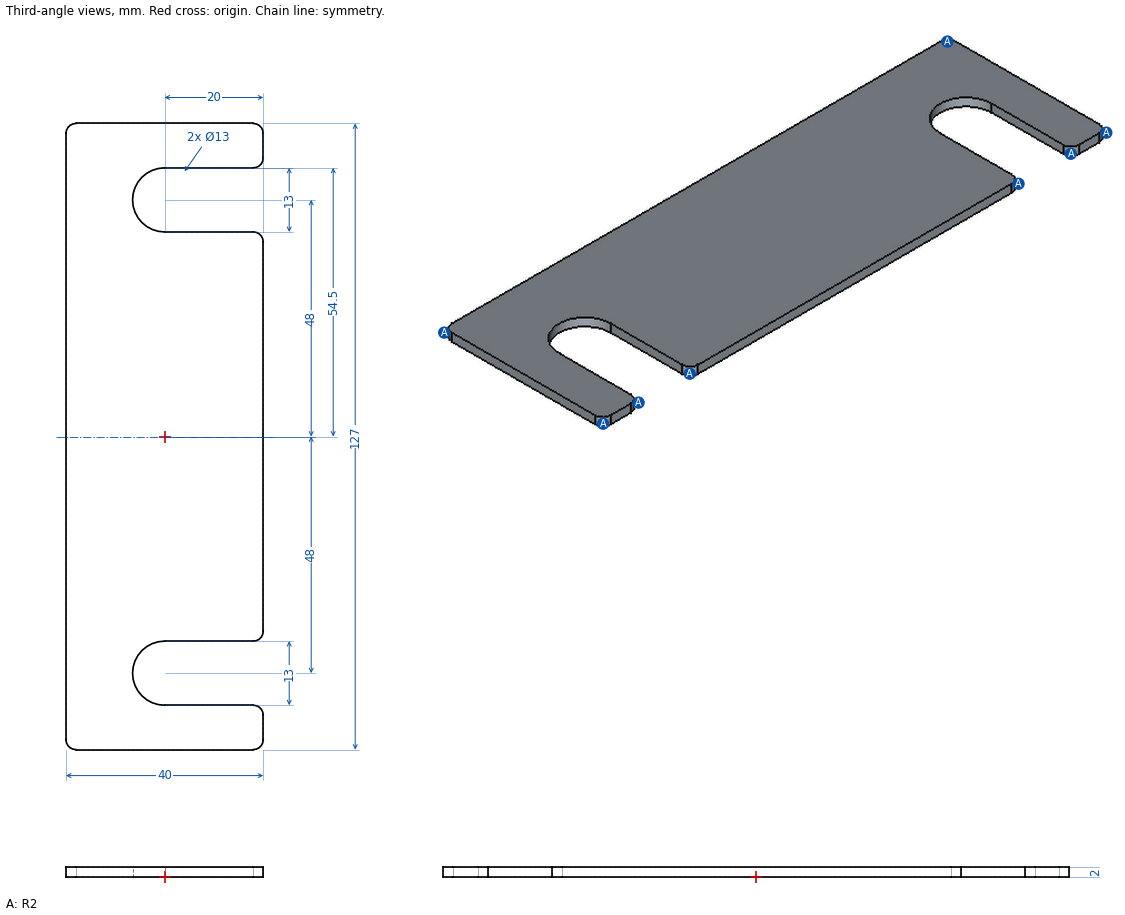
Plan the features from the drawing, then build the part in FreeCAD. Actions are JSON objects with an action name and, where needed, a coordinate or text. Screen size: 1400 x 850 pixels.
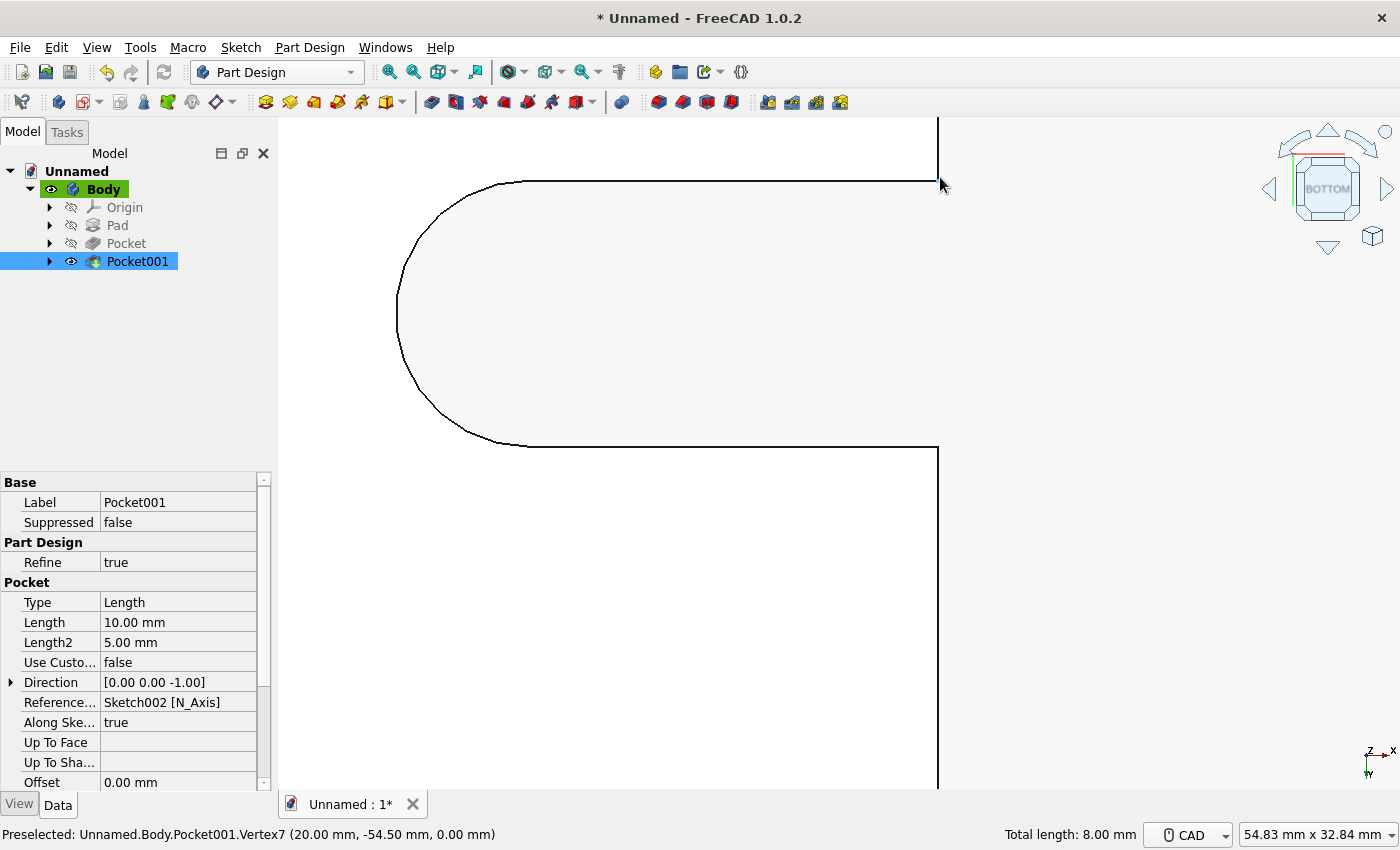
{"action": "left_click", "coordinate": [390, 72]}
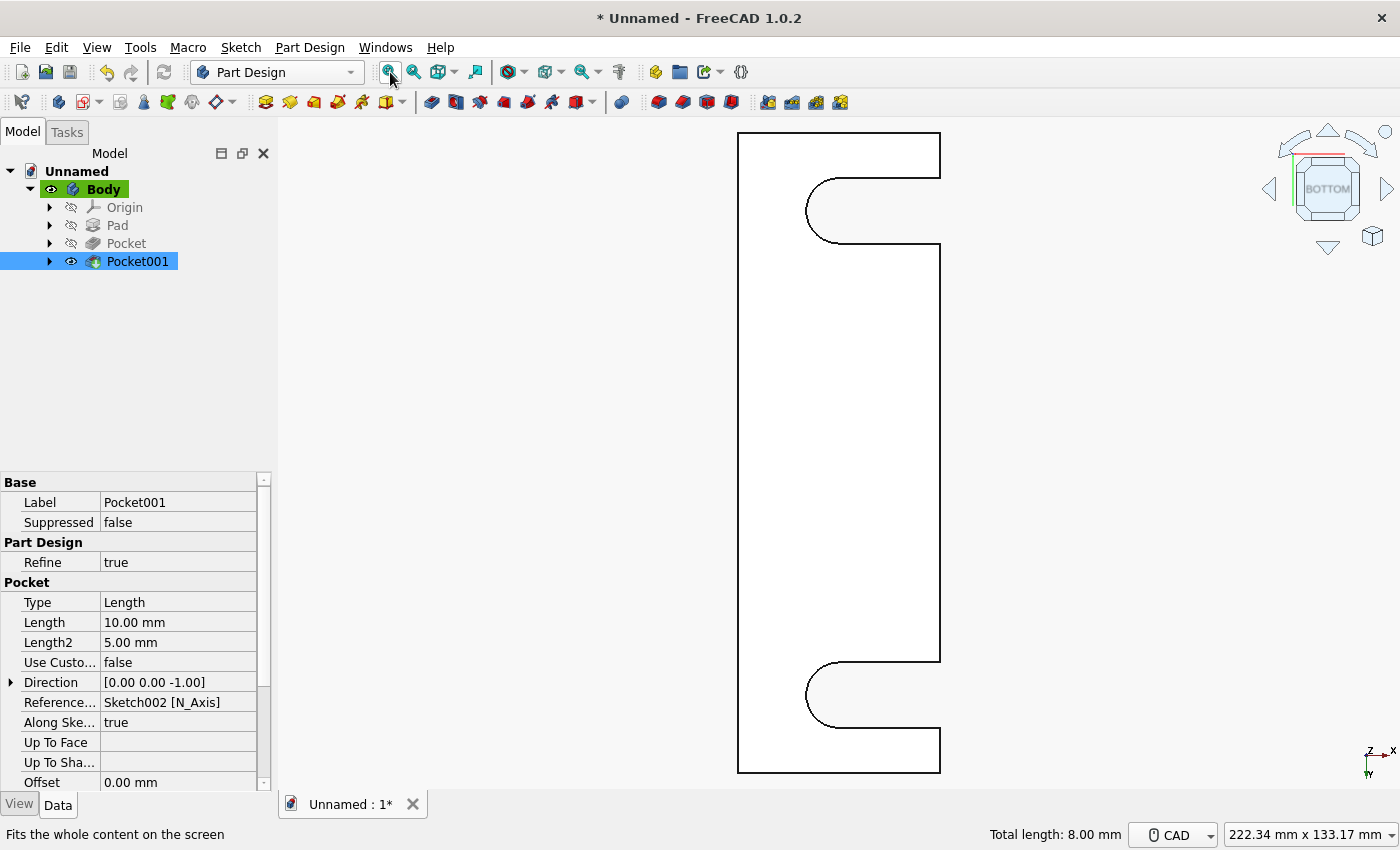
{"action": "key", "text": "4"}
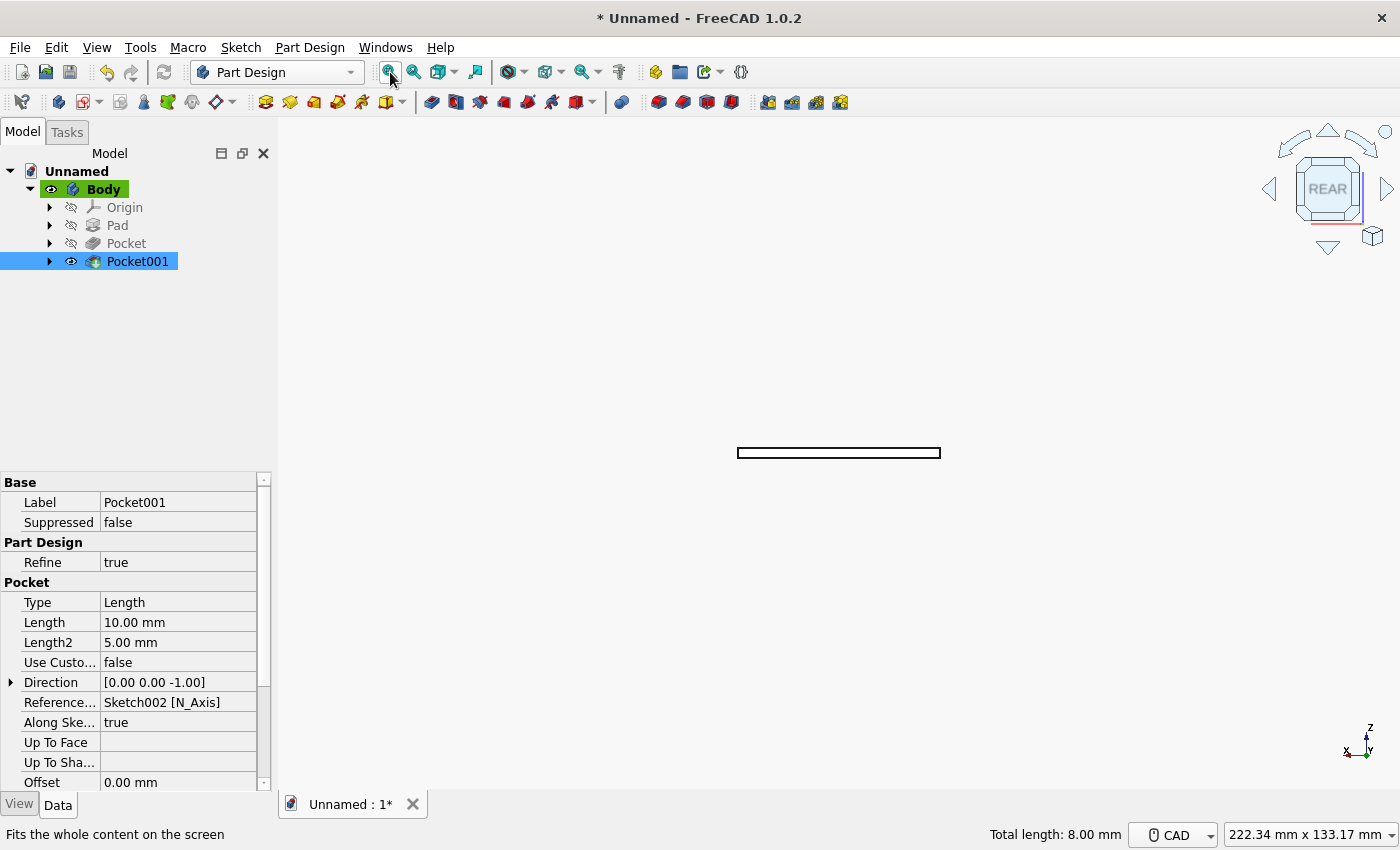
{"action": "left_click", "coordinate": [390, 72]}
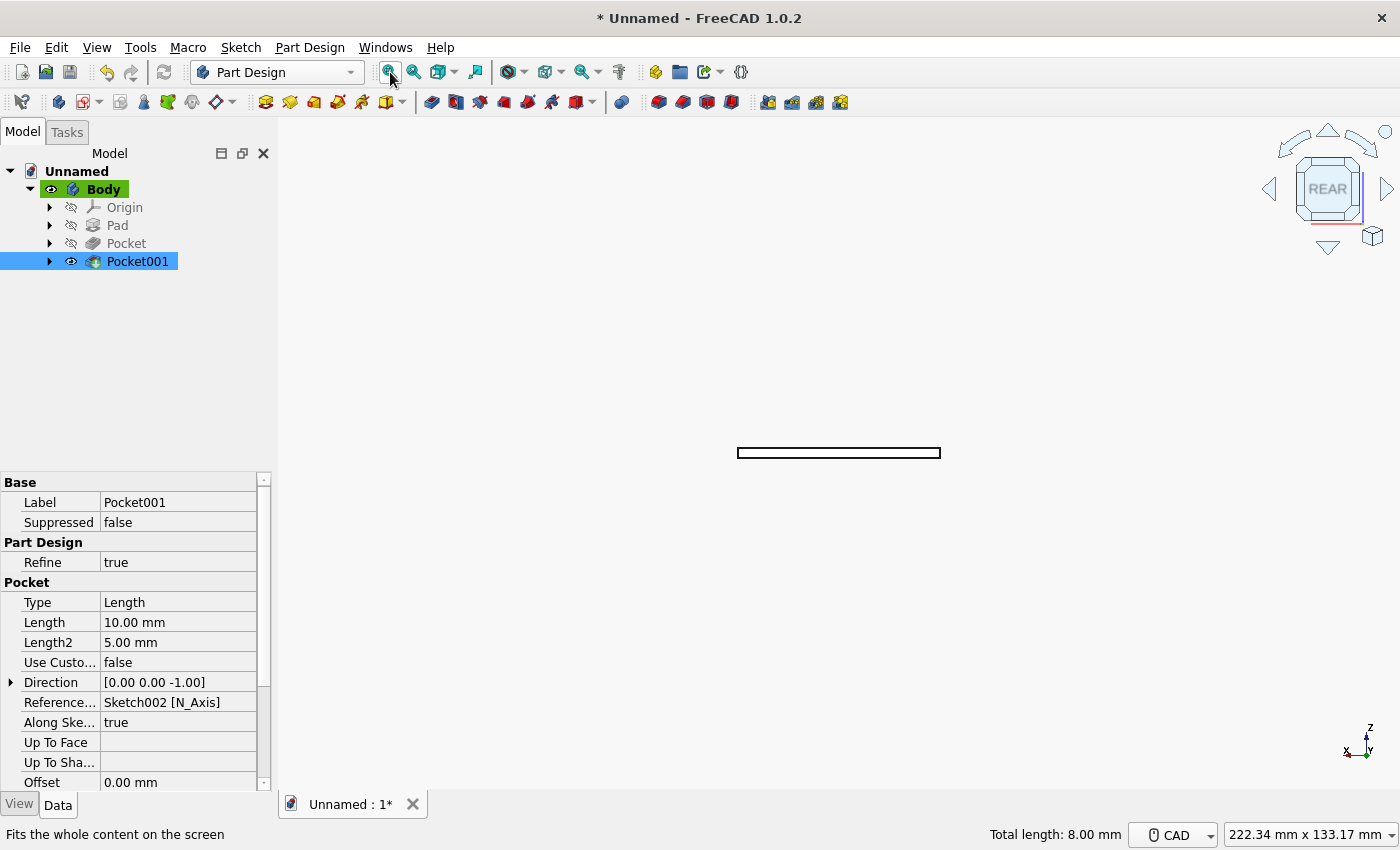
{"action": "scroll", "coordinate": [738, 452], "scroll_direction": "up", "scroll_amount": 7}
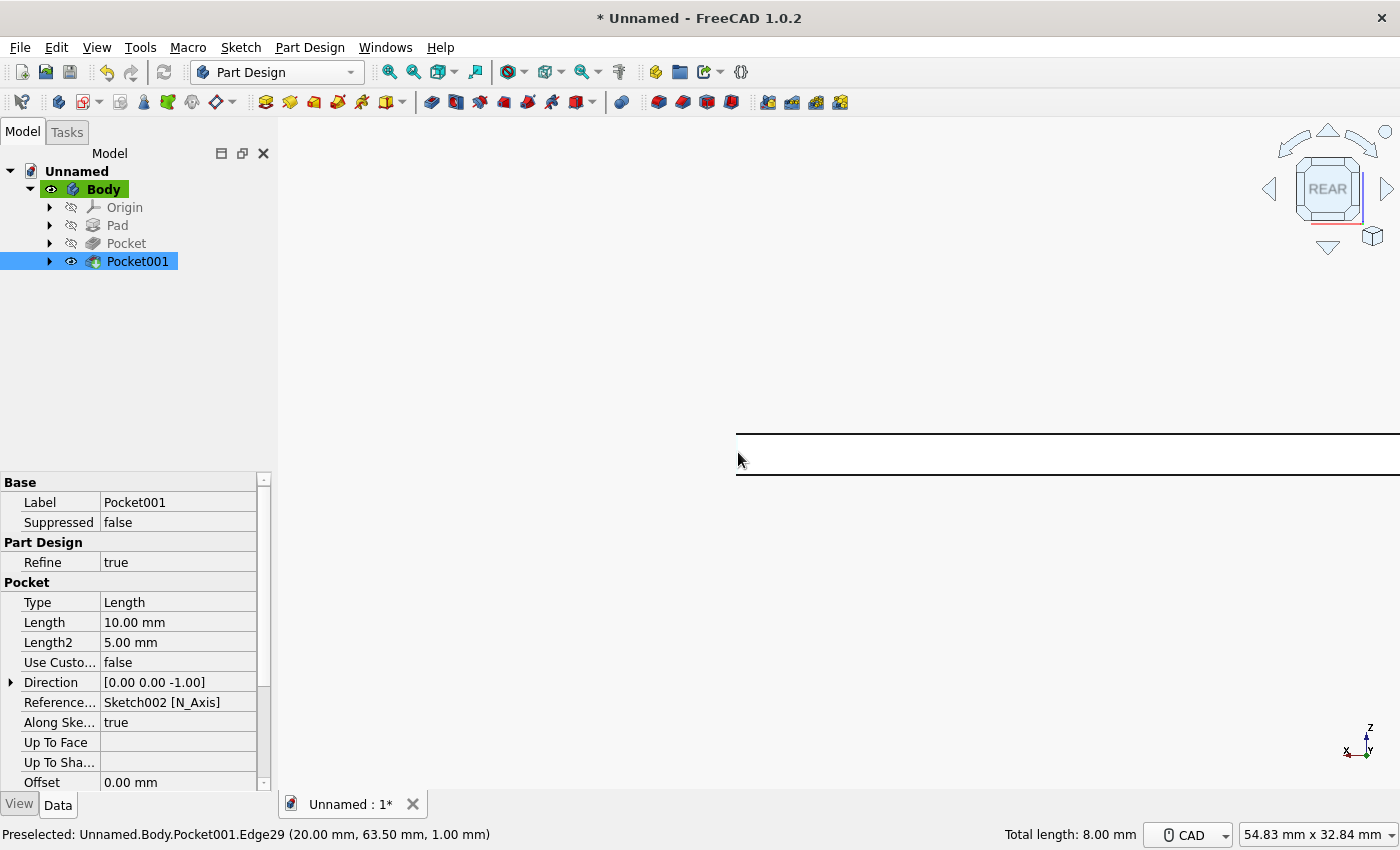
{"action": "left_click", "coordinate": [737, 454], "text": "ctrl"}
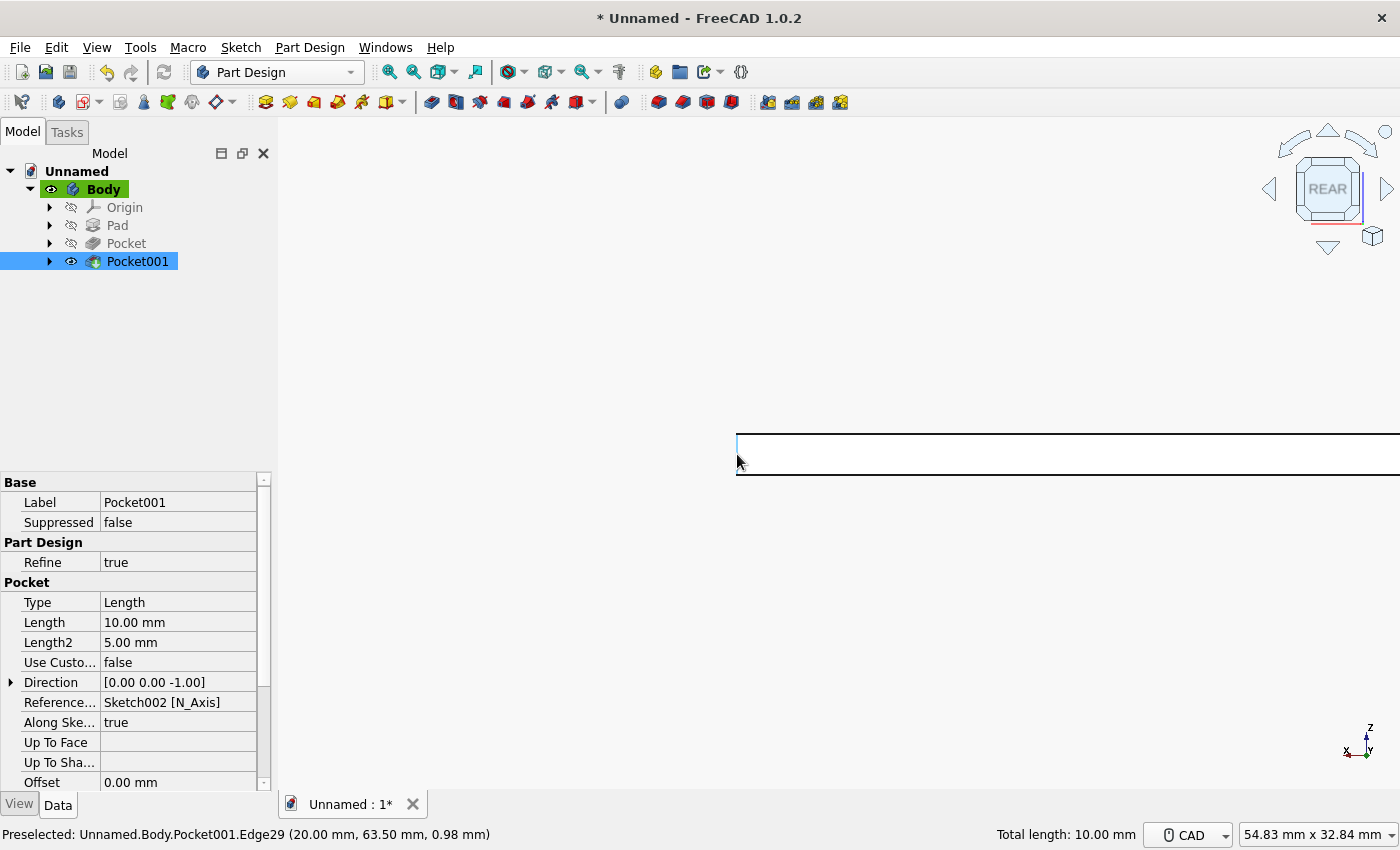
{"action": "left_click", "coordinate": [390, 72]}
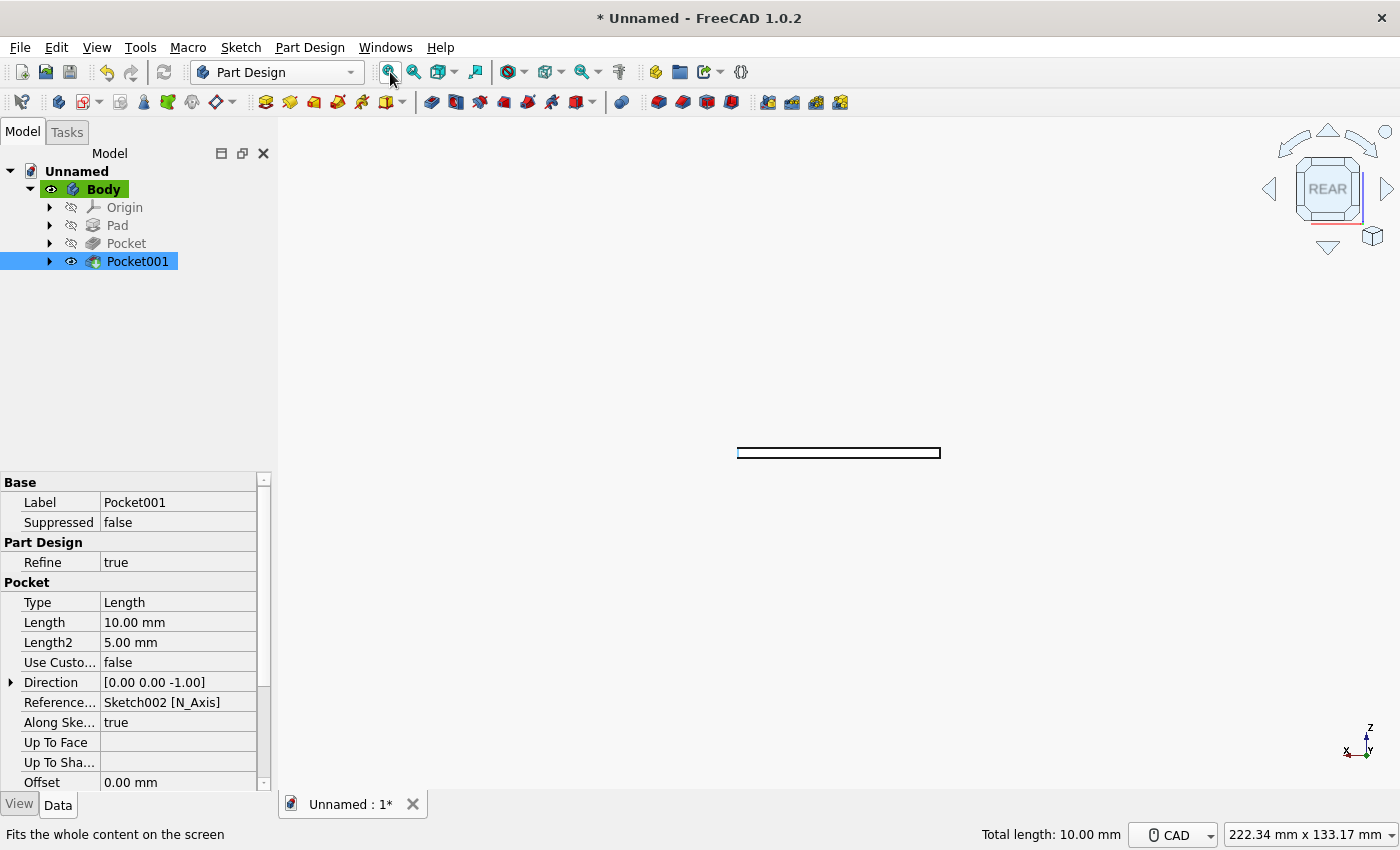
{"action": "key", "text": "6"}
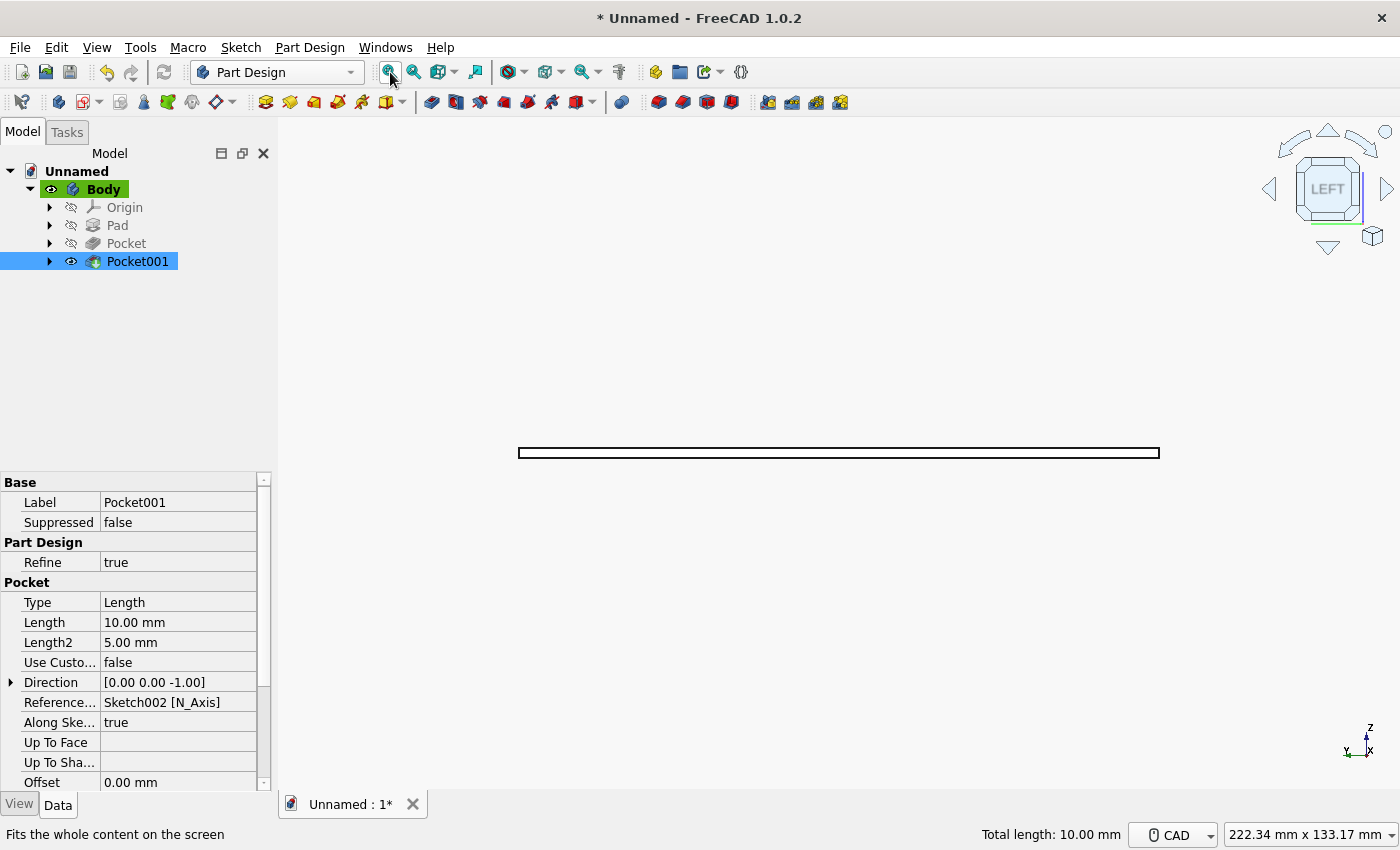
{"action": "scroll", "coordinate": [1114, 452], "scroll_direction": "up", "scroll_amount": 7}